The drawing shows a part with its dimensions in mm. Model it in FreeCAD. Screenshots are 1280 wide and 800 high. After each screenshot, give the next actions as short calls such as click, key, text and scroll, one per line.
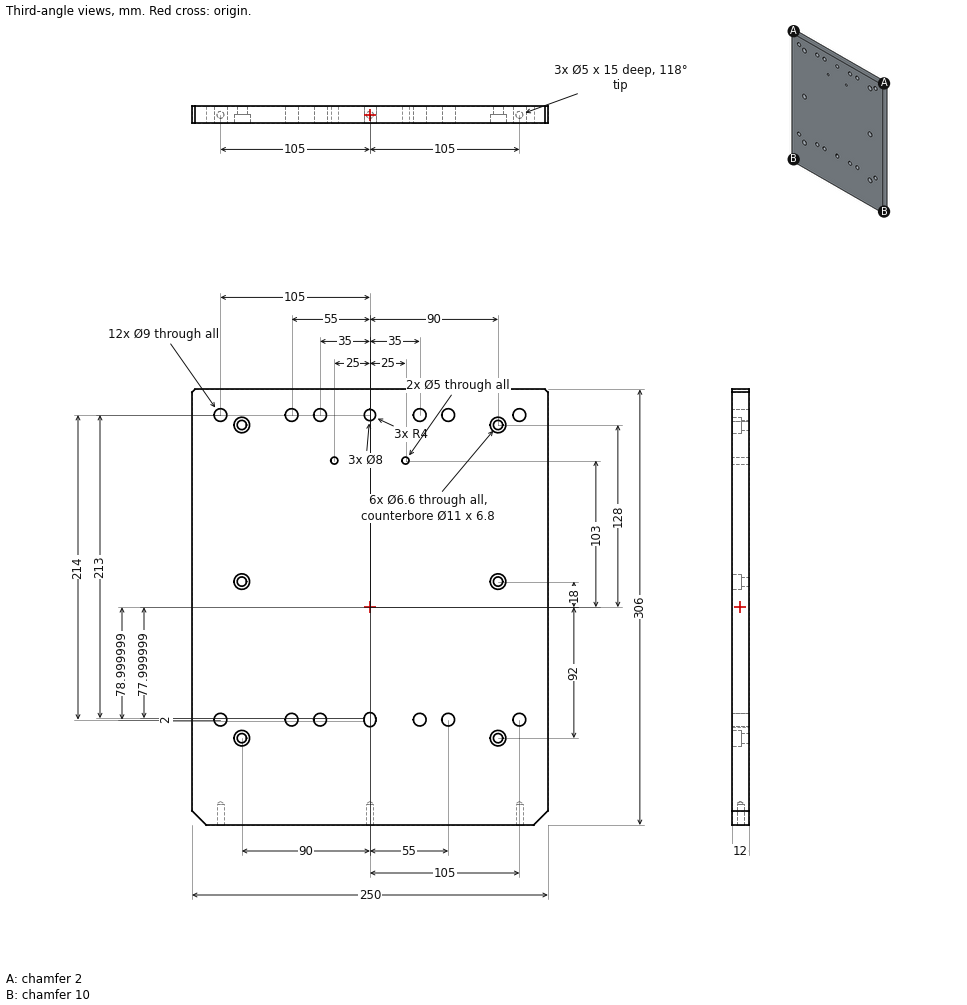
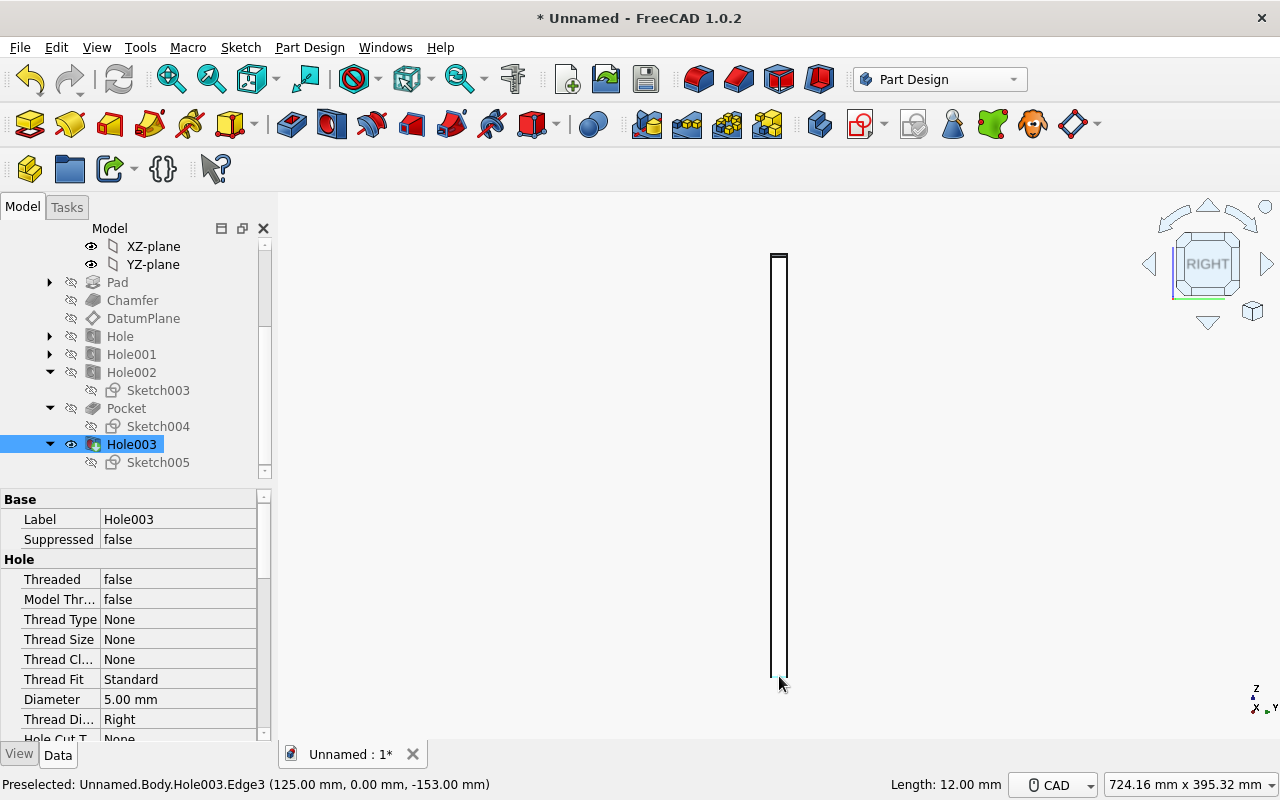
key(5)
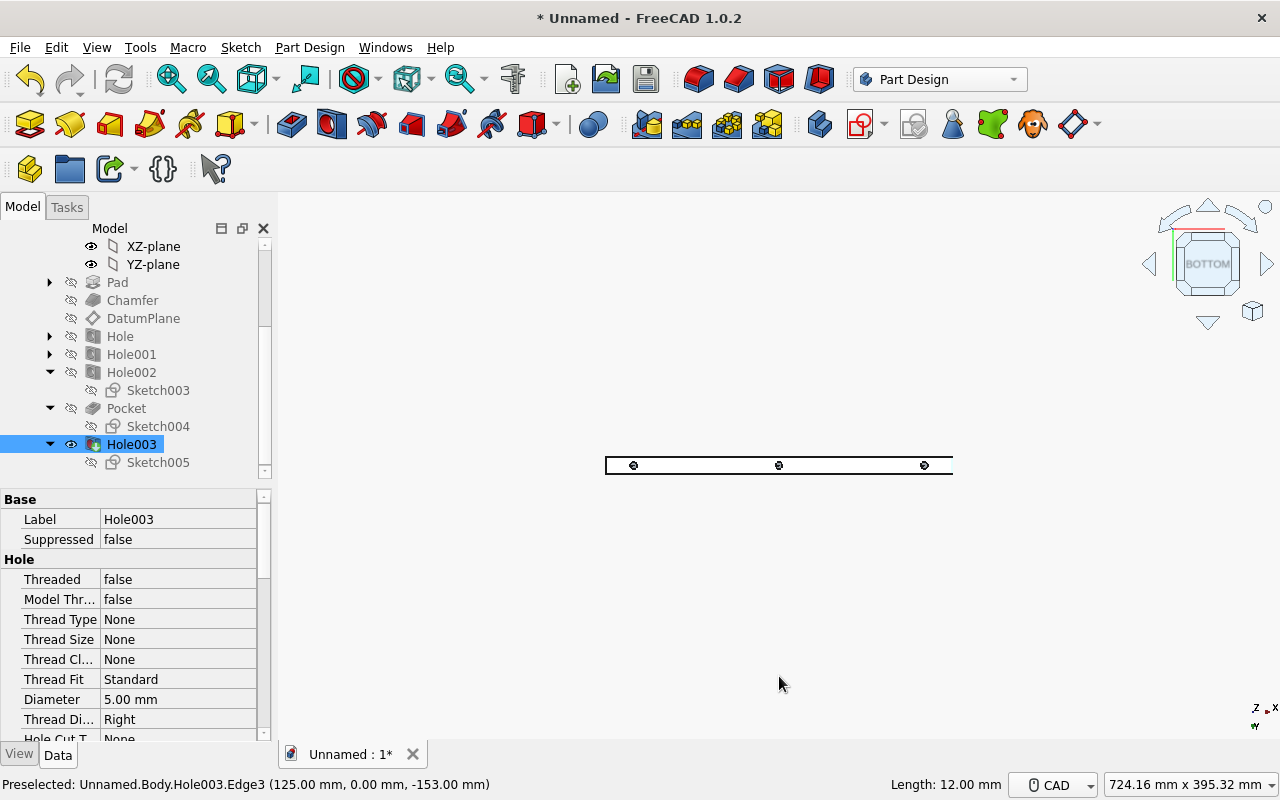
click(172, 80)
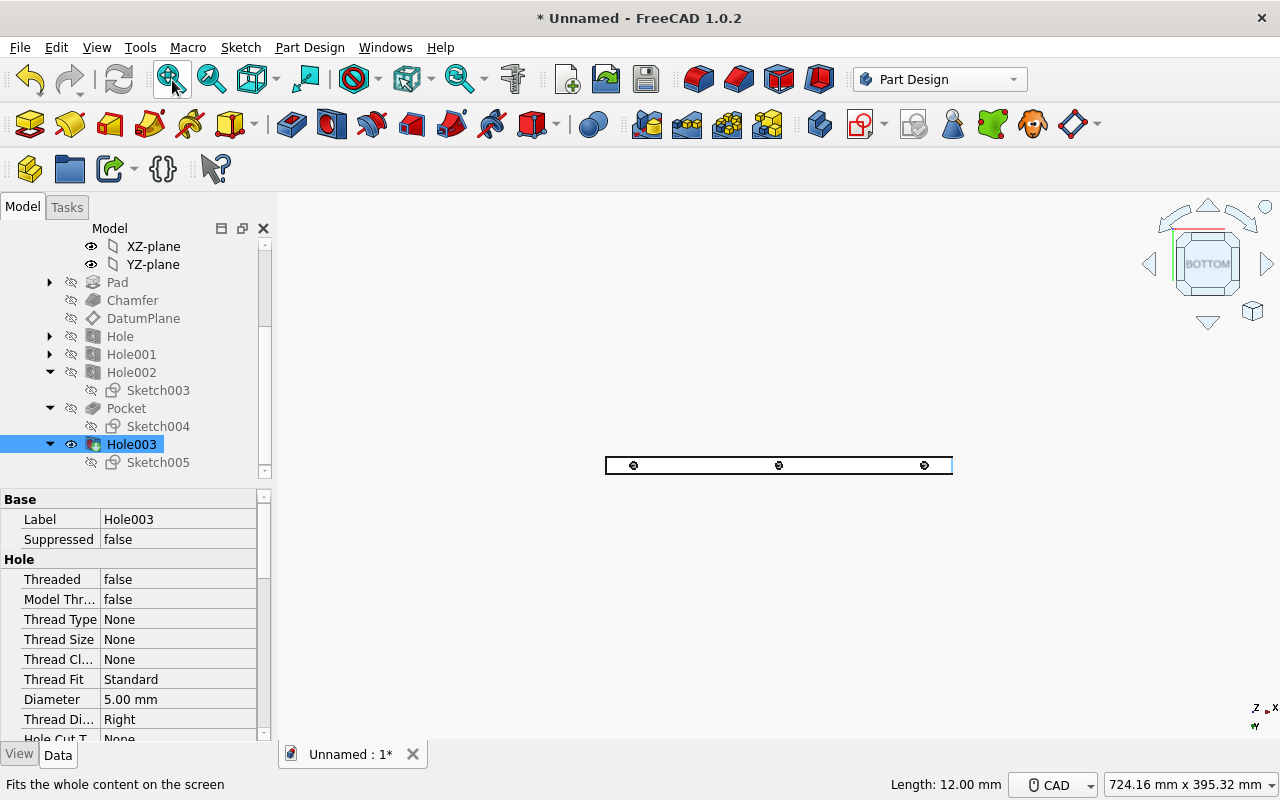
click(606, 464, ctrl)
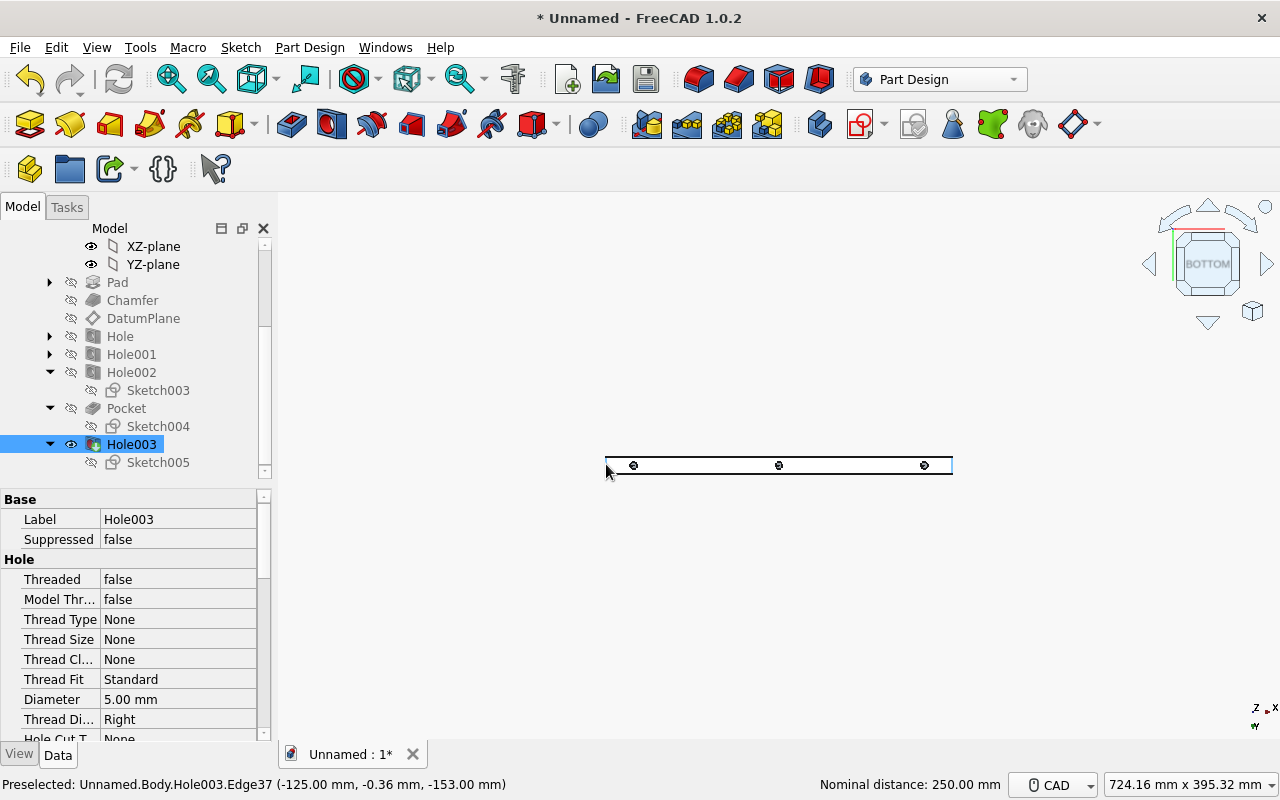
click(740, 80)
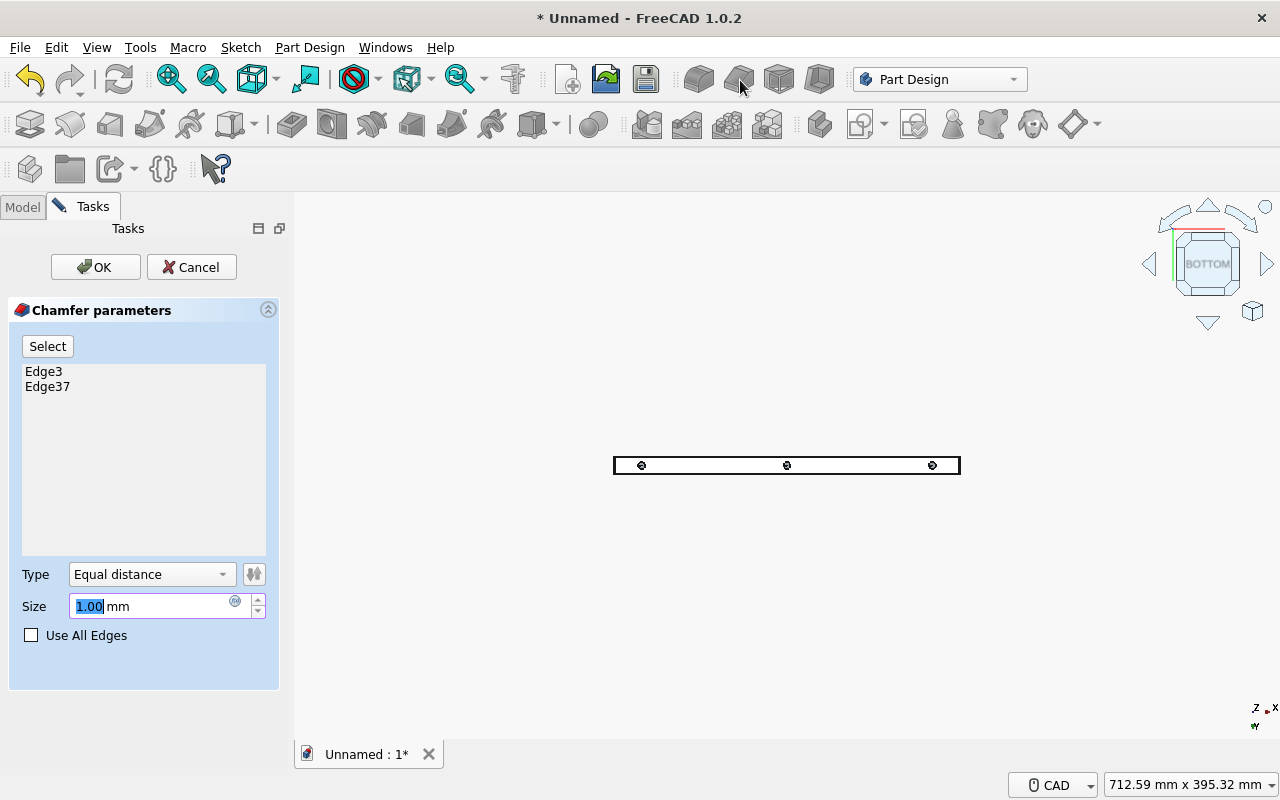
text(10)
key(Tab)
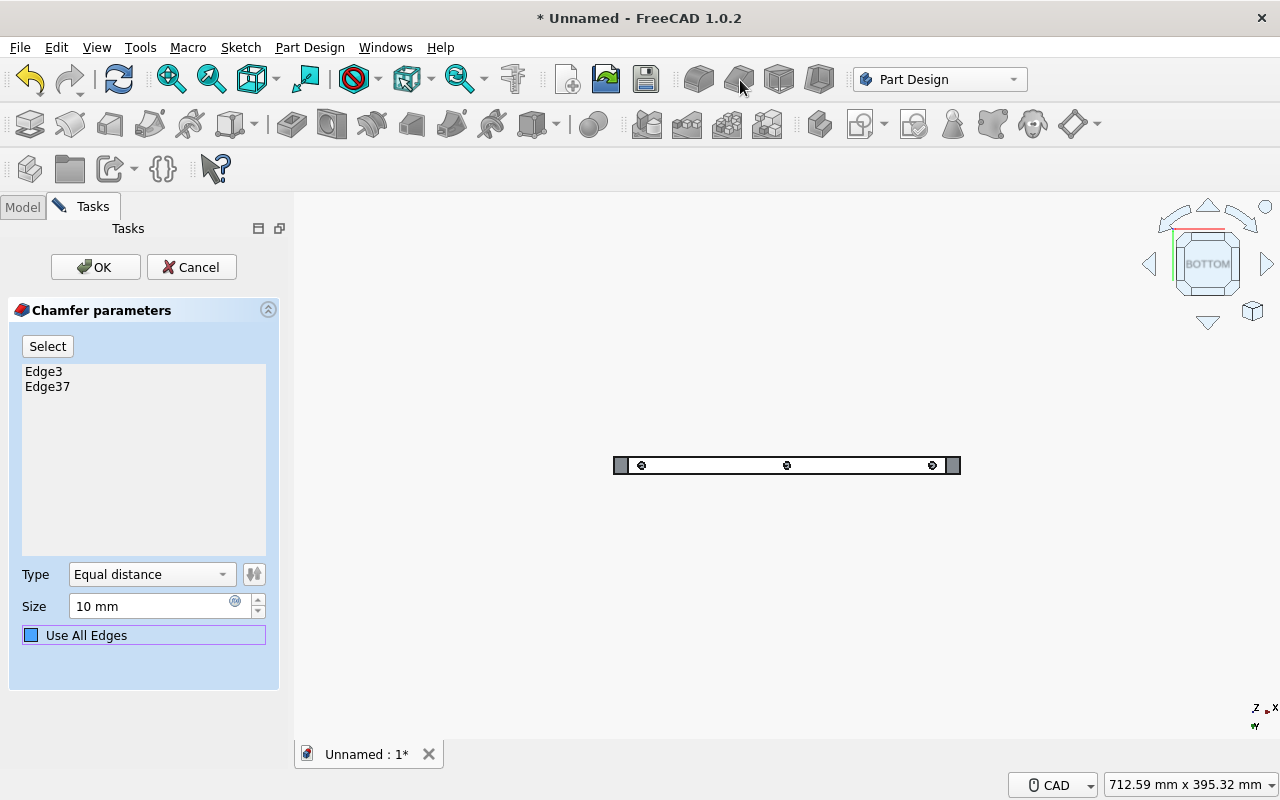
click(96, 267)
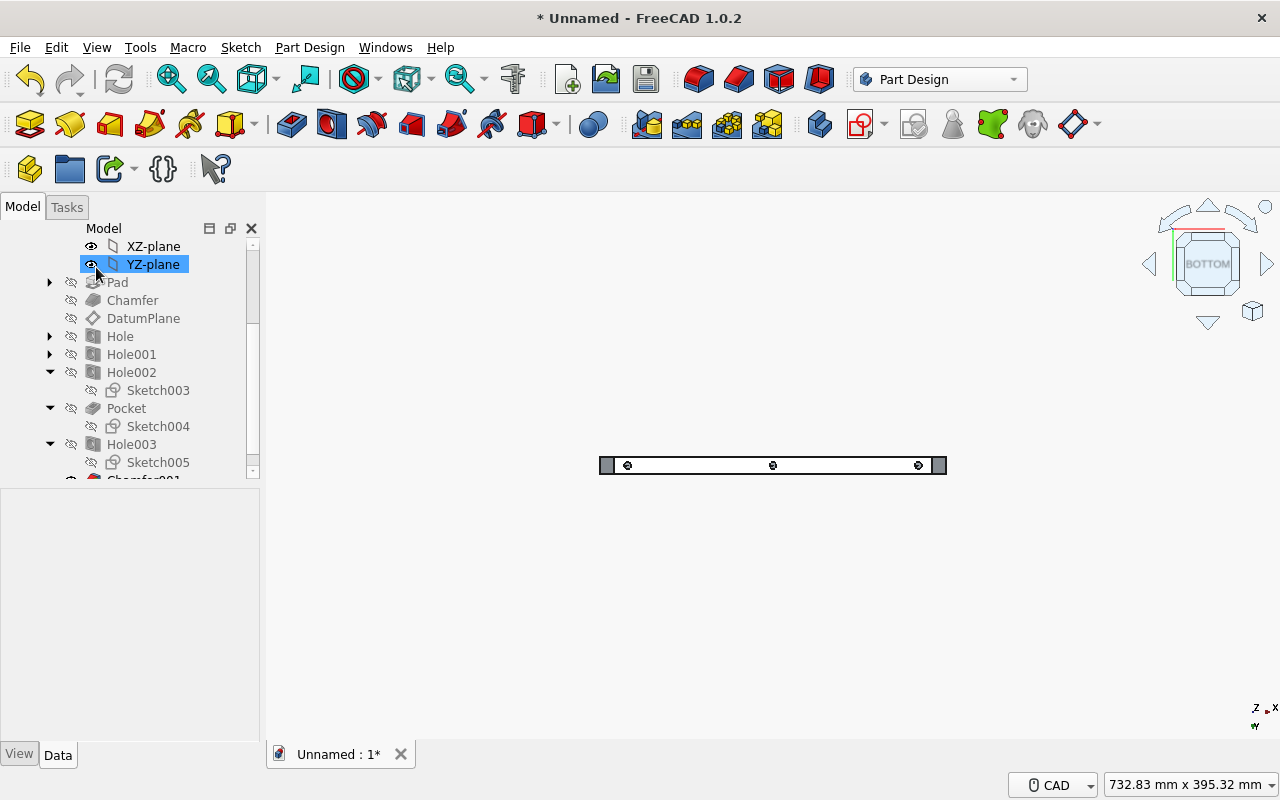
key(0)